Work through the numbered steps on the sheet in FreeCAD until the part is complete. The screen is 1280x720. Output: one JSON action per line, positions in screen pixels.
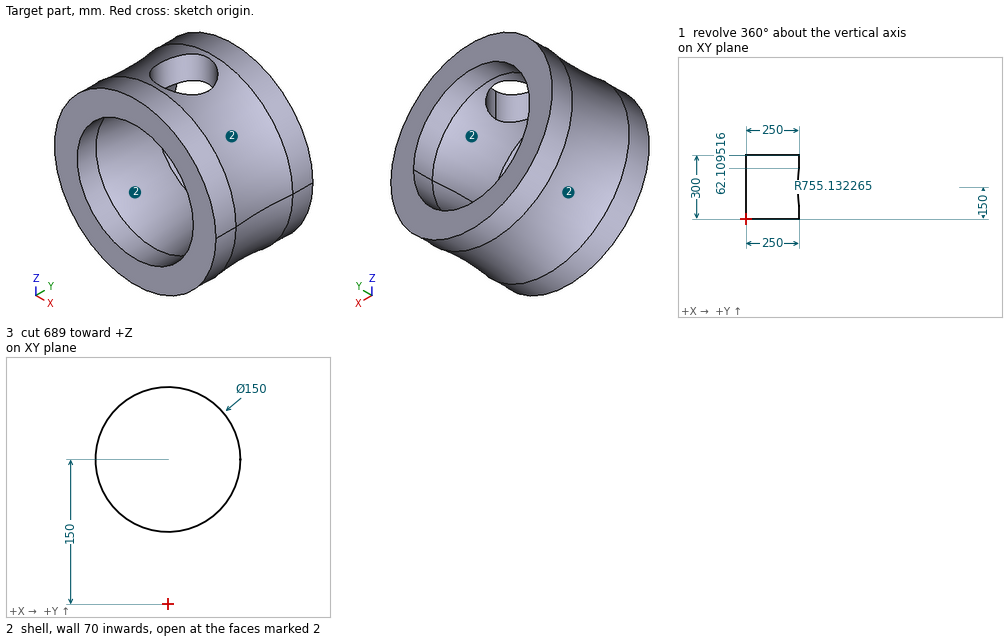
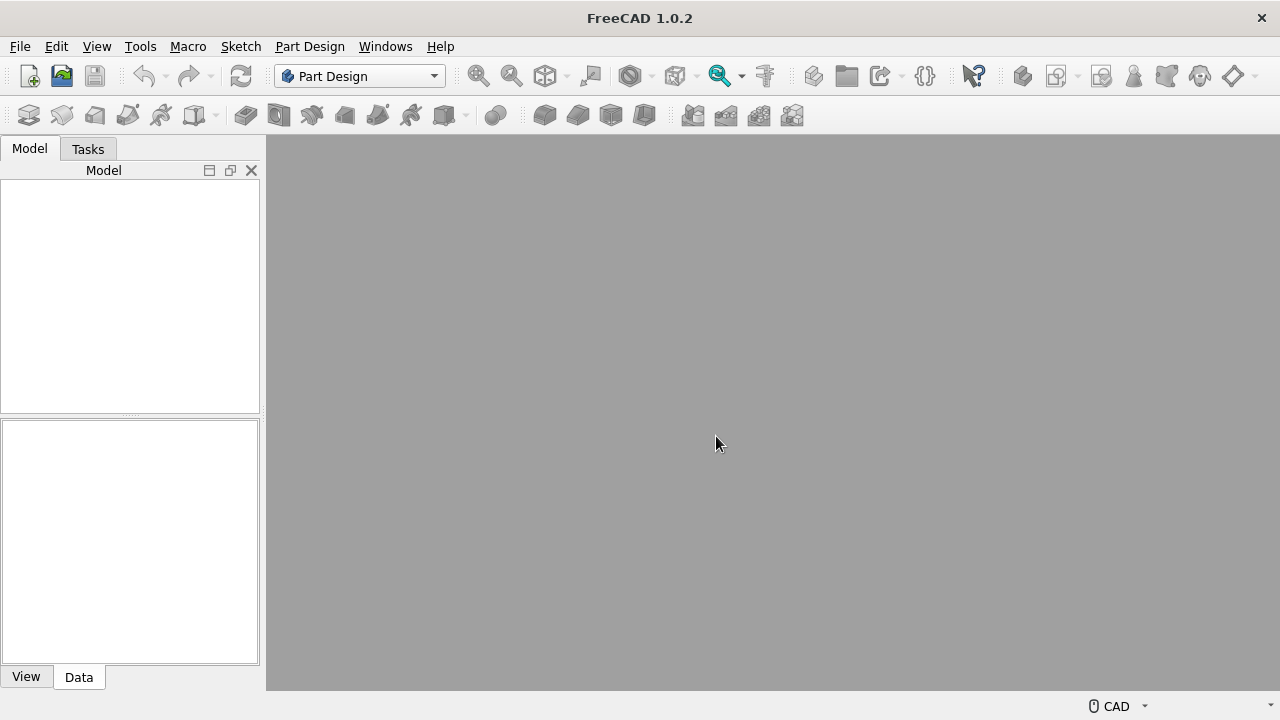
{"action": "left_click", "coordinate": [29, 76]}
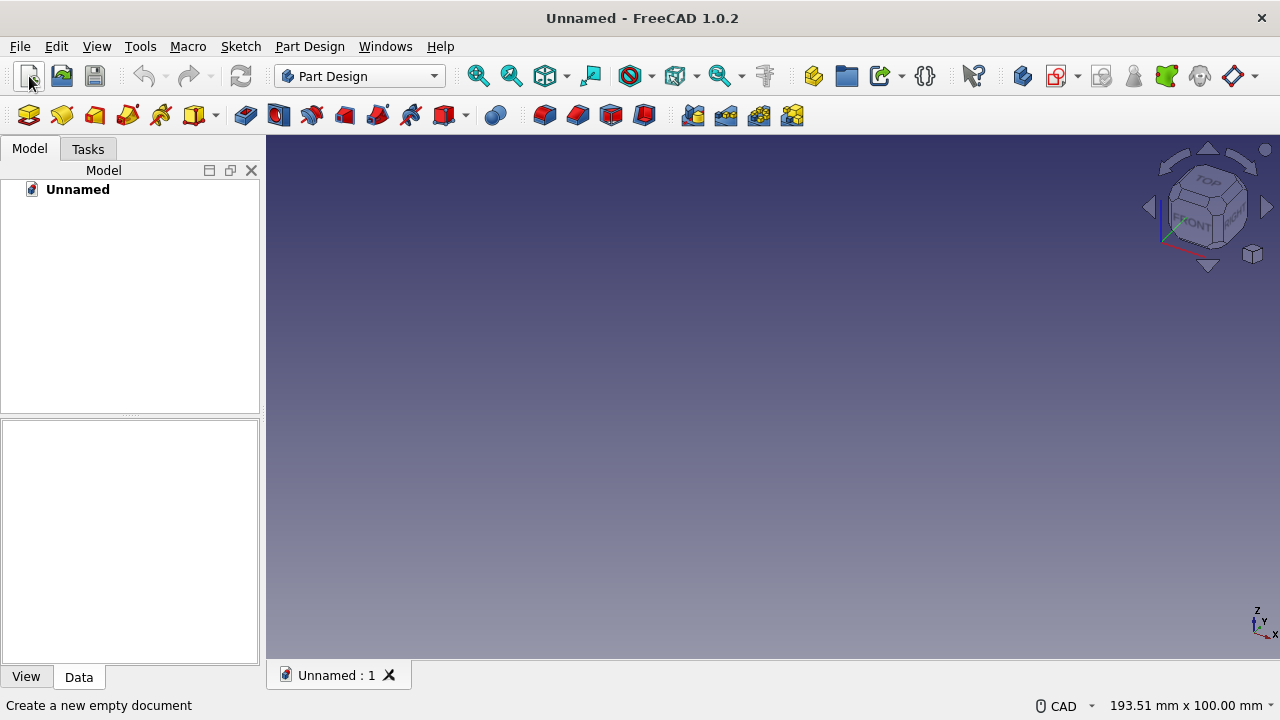
{"action": "left_click", "coordinate": [1056, 76]}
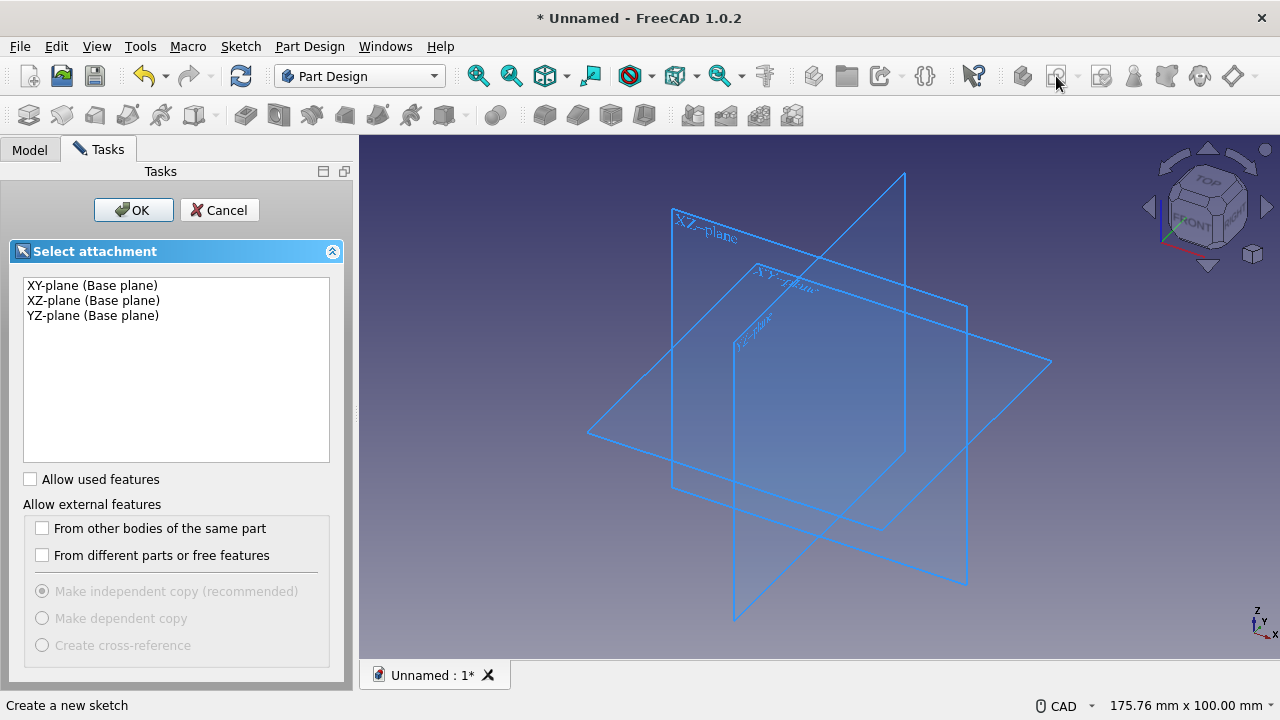
{"action": "left_click", "coordinate": [84, 286]}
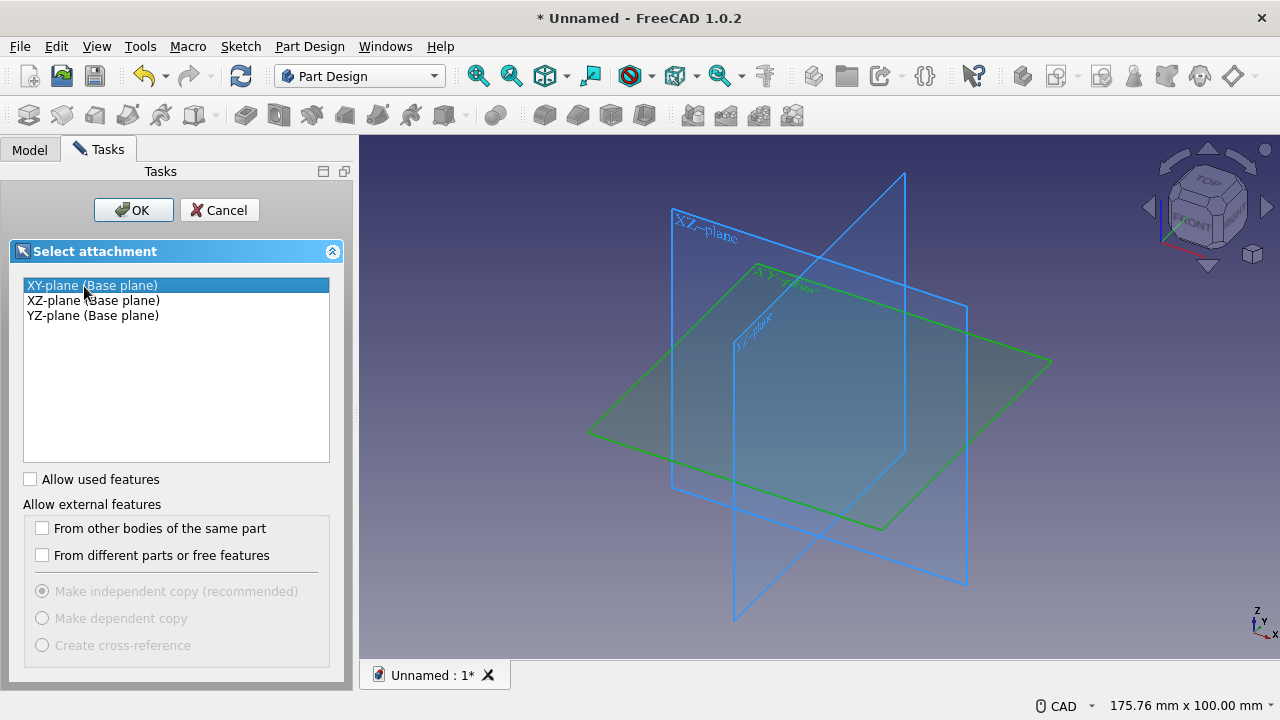
{"action": "left_click", "coordinate": [134, 210]}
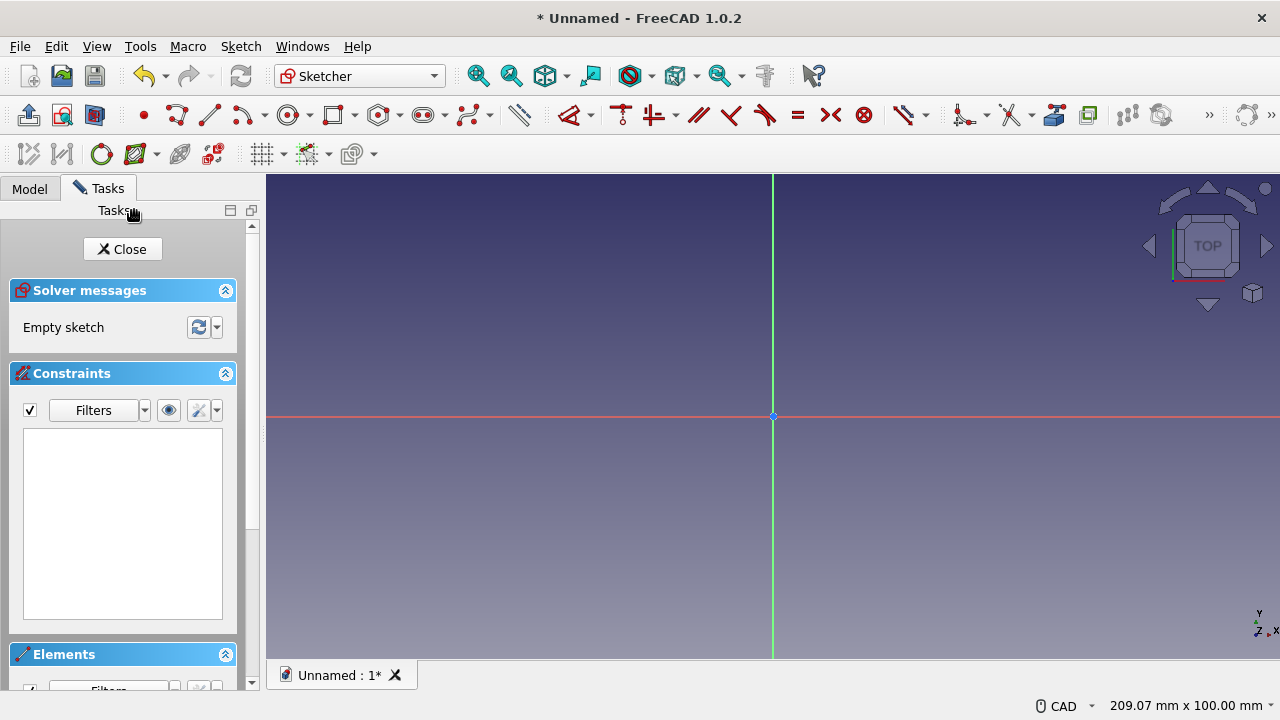
{"action": "scroll", "coordinate": [534, 601], "scroll_direction": "down", "scroll_amount": 8}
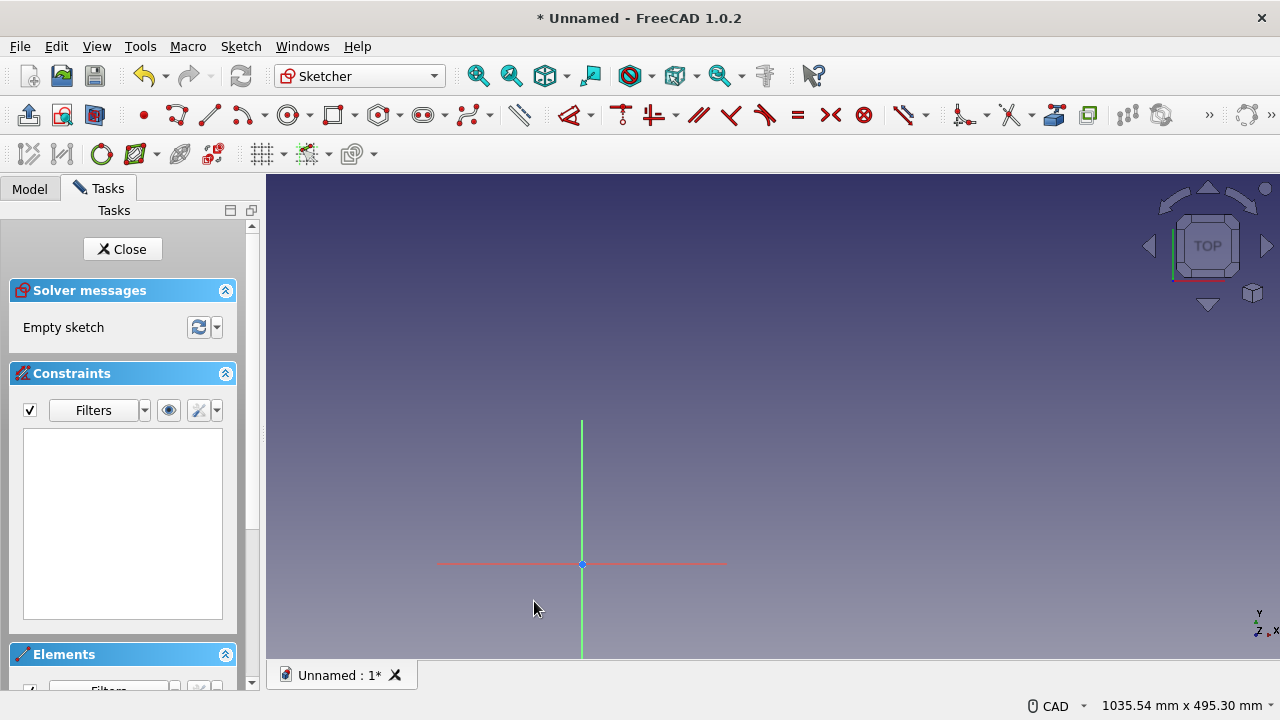
{"action": "left_click", "coordinate": [177, 116]}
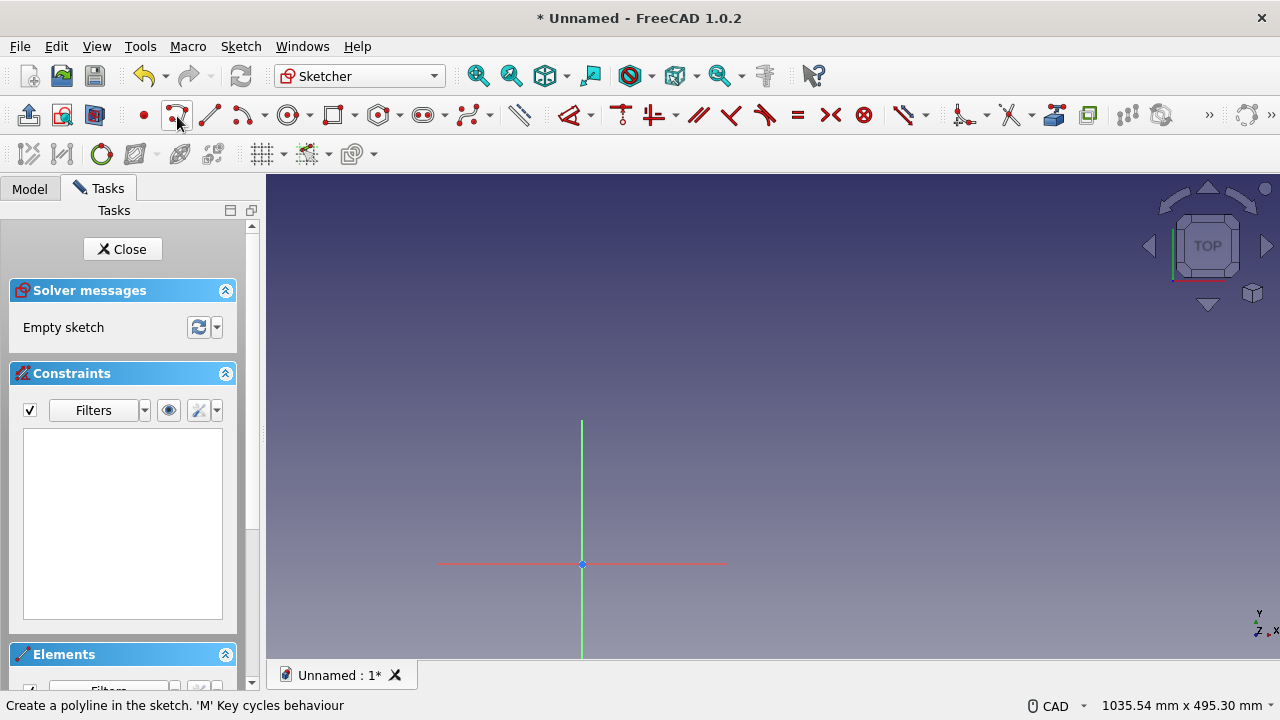
{"action": "left_click", "coordinate": [827, 332]}
{"action": "left_click", "coordinate": [827, 271]}
{"action": "left_click", "coordinate": [582, 271]}
{"action": "left_click", "coordinate": [582, 564]}
{"action": "left_click", "coordinate": [827, 555]}
{"action": "left_click", "coordinate": [827, 504]}
{"action": "right_click", "coordinate": [827, 504]}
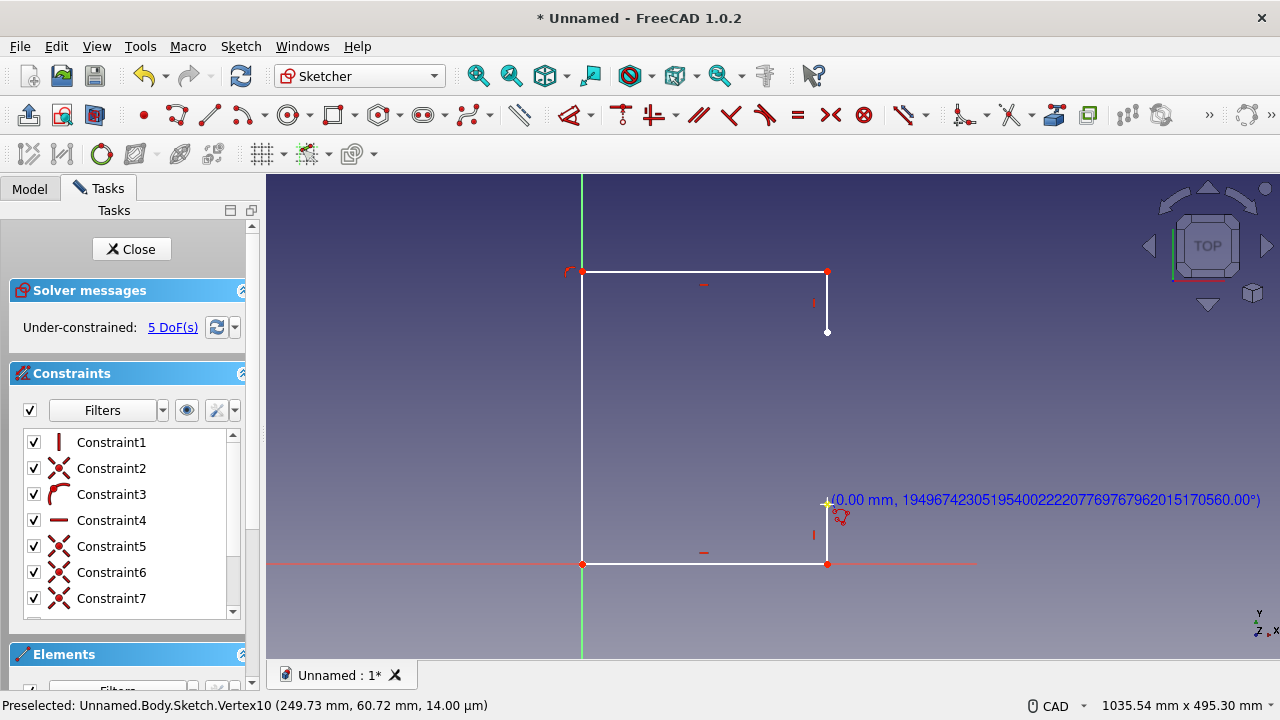
{"action": "key", "text": "g 3 a"}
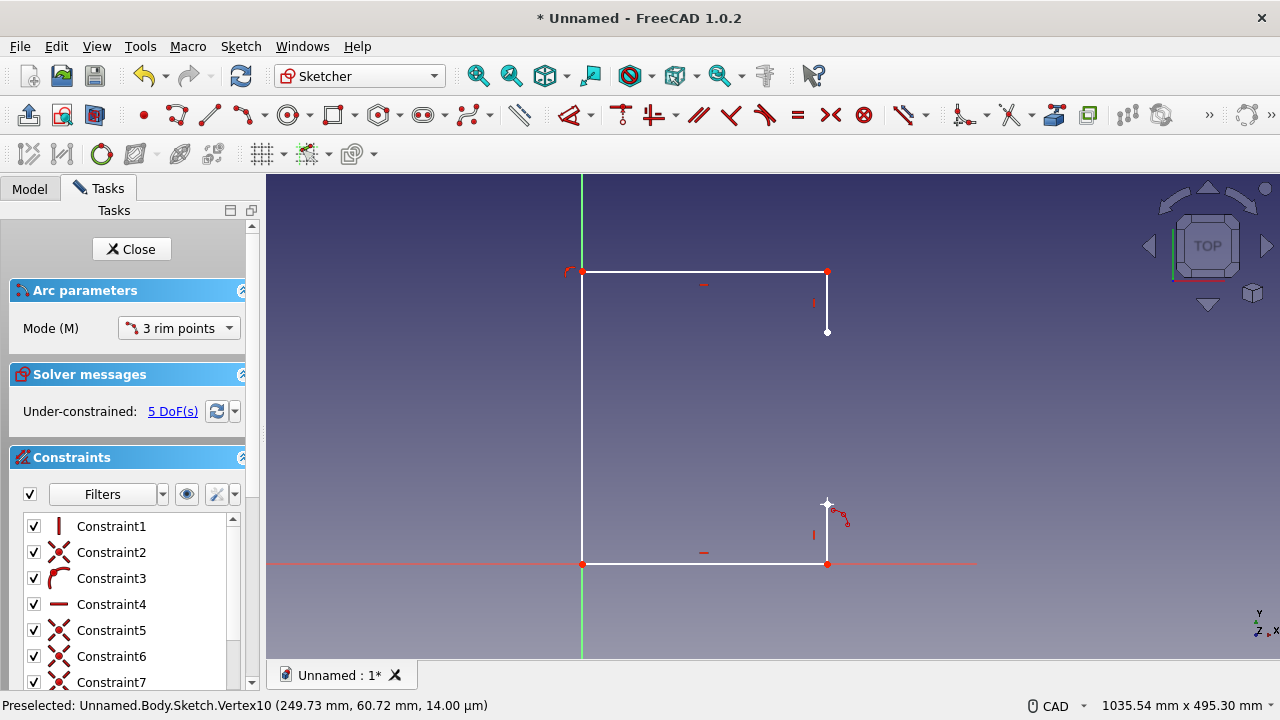
{"action": "left_click", "coordinate": [827, 505]}
{"action": "left_click", "coordinate": [827, 333]}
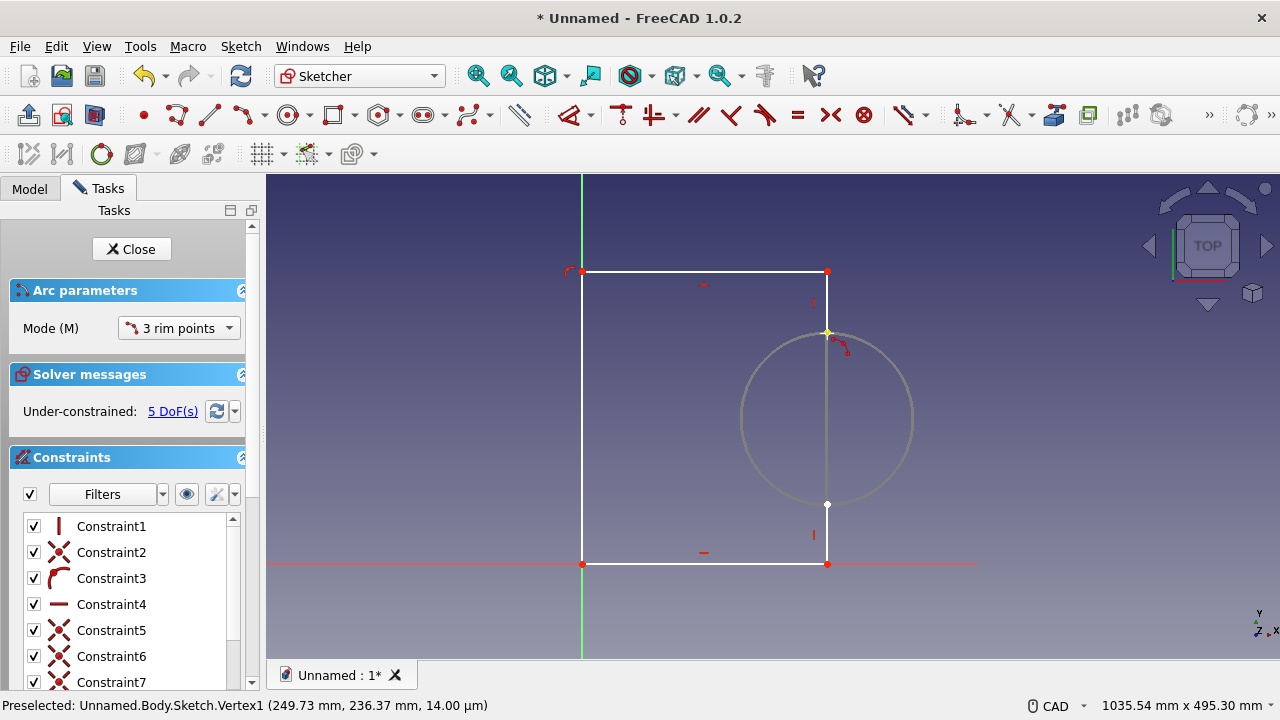
{"action": "scroll", "coordinate": [822, 418], "scroll_direction": "up", "scroll_amount": 6}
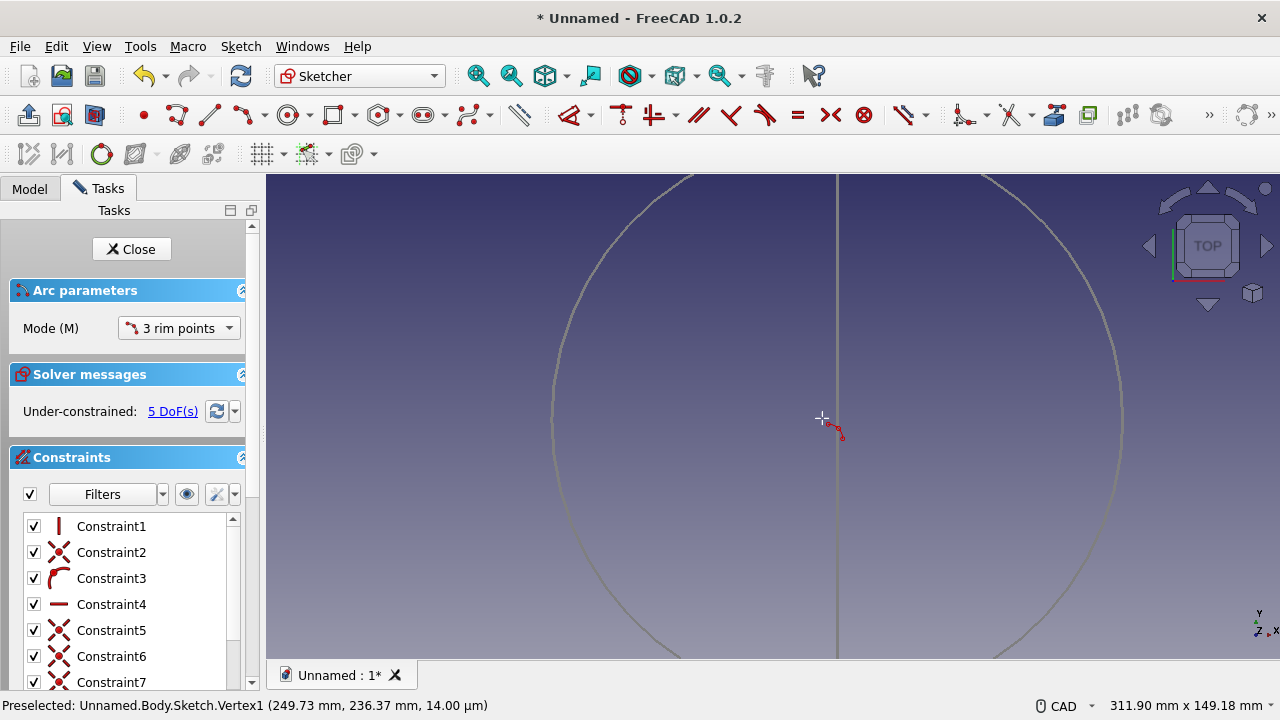
{"action": "left_click", "coordinate": [822, 415]}
{"action": "key", "text": "Escape"}